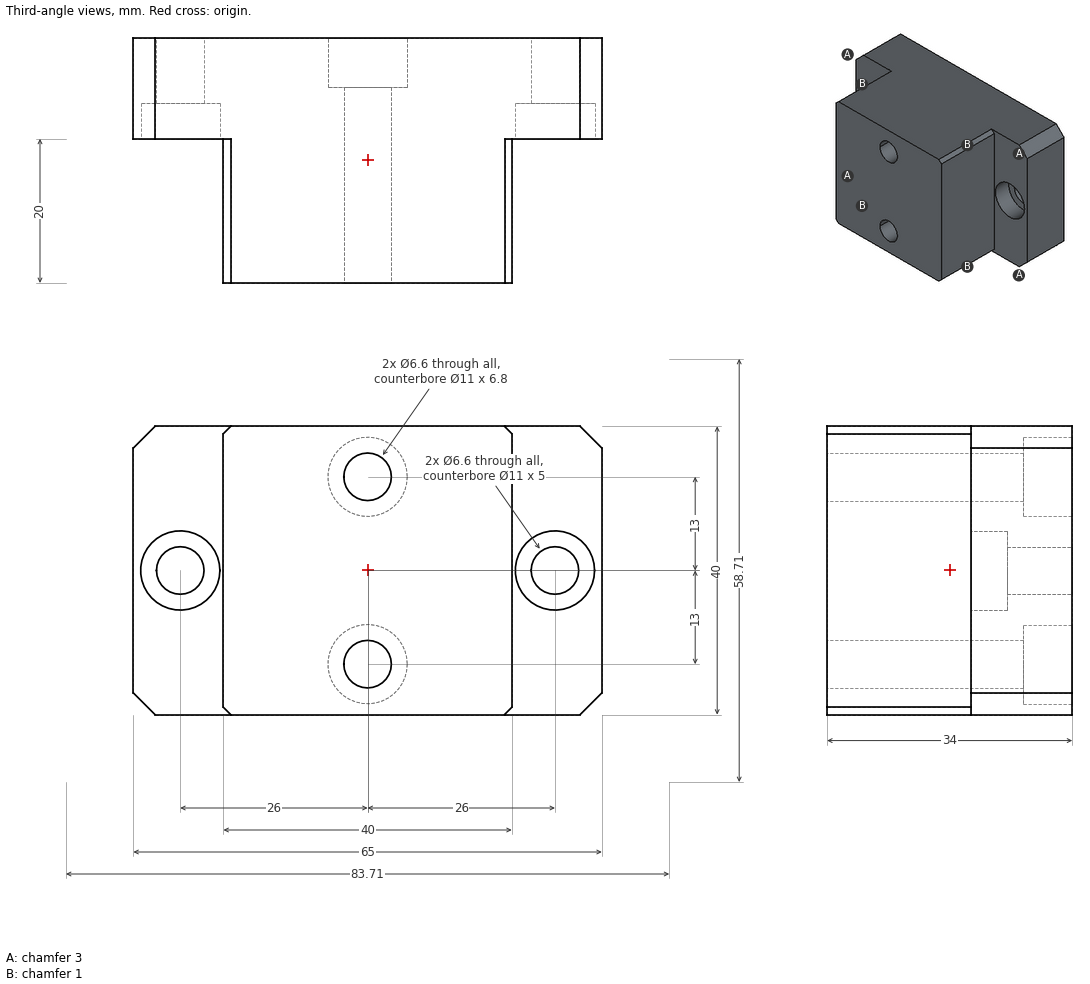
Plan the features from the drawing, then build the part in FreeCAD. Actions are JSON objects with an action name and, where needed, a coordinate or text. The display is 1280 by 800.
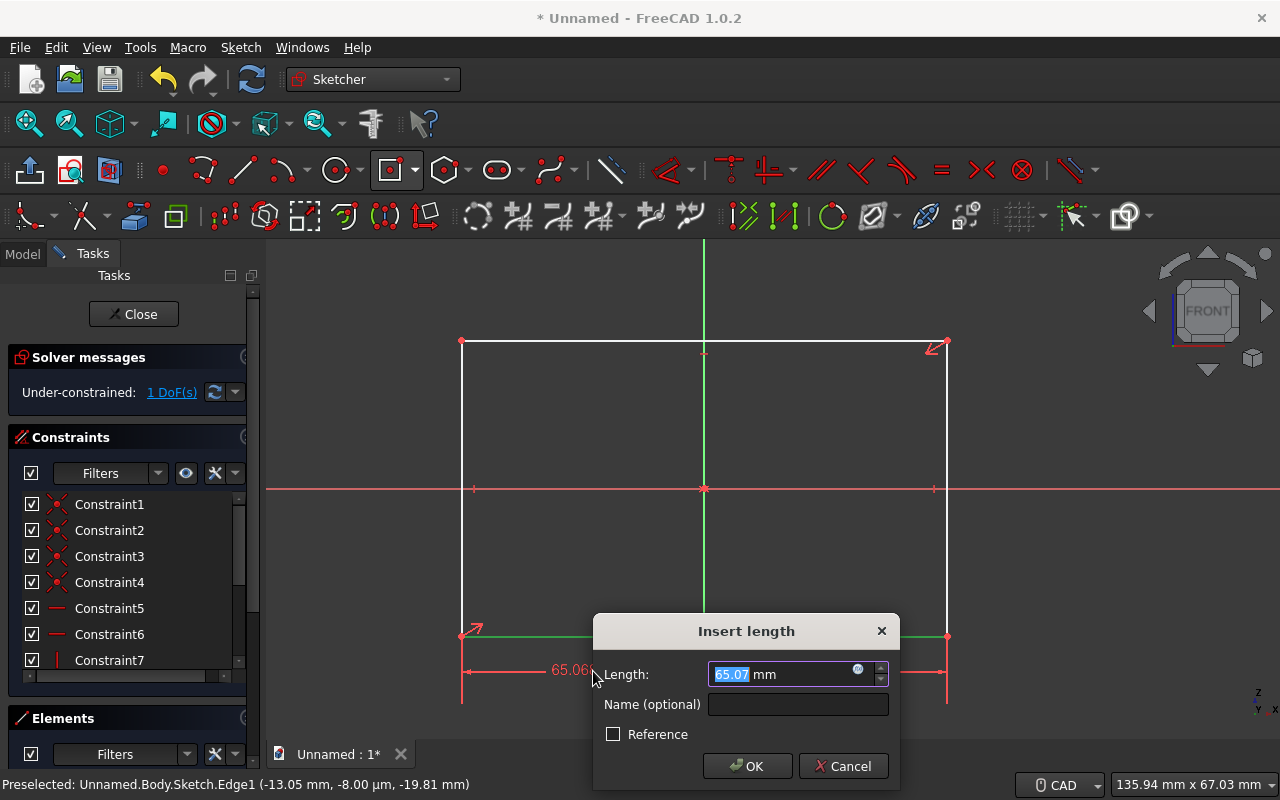
{"action": "type", "text": "65"}
{"action": "key", "text": "Return"}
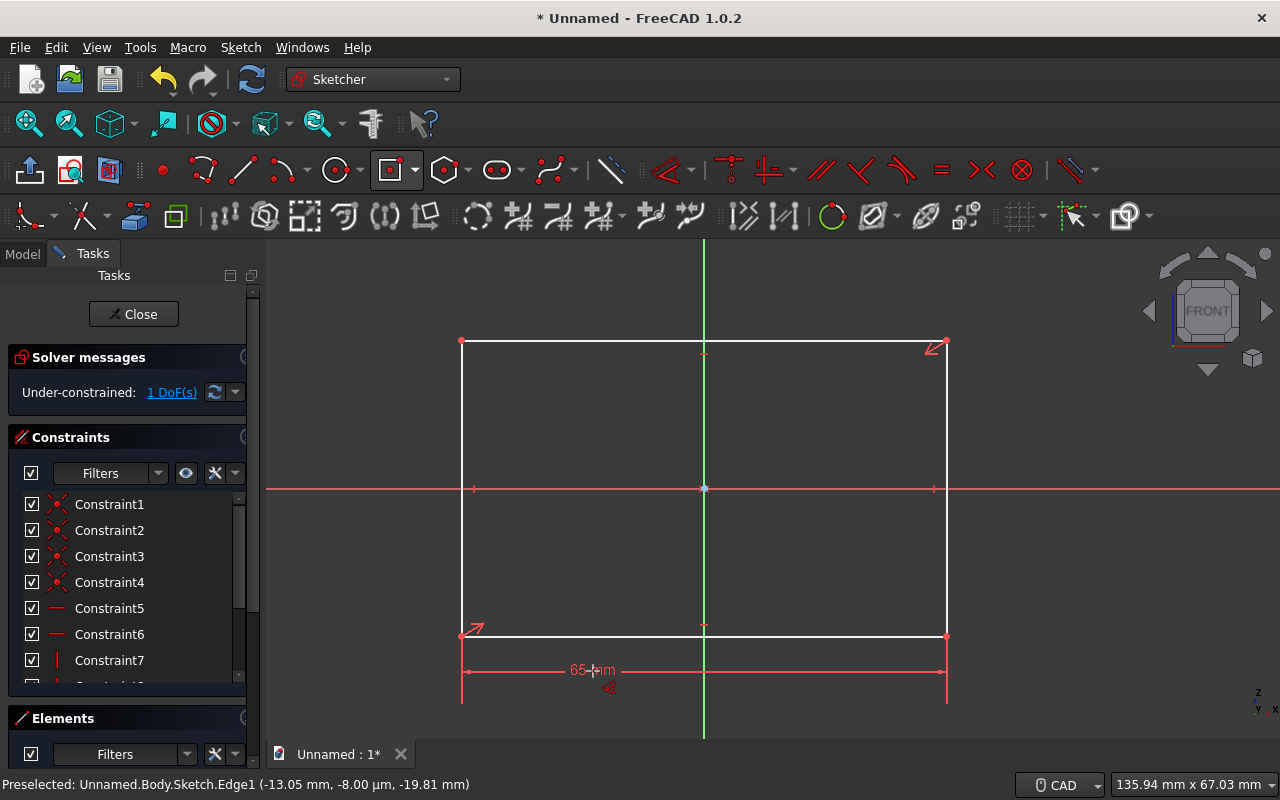
{"action": "left_click", "coordinate": [947, 548]}
{"action": "left_click", "coordinate": [981, 421]}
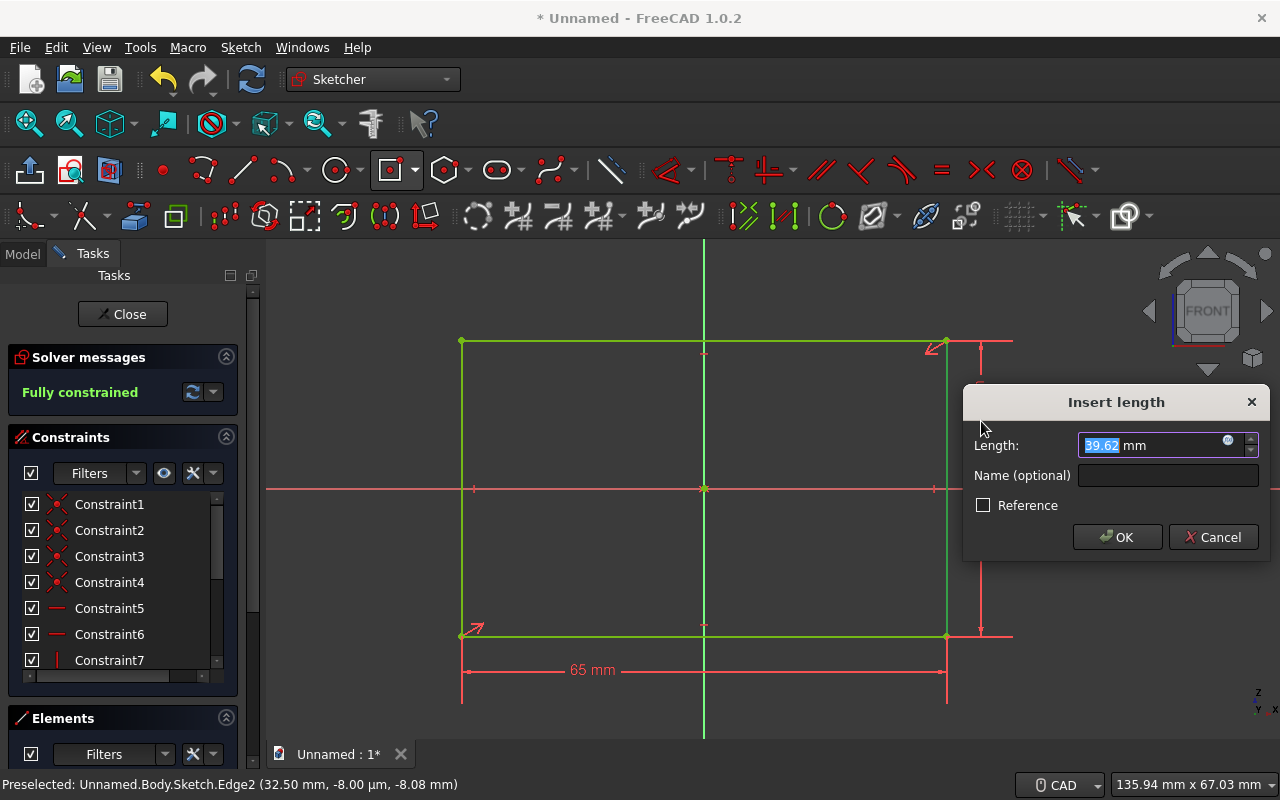
{"action": "type", "text": "40"}
{"action": "key", "text": "Return"}
{"action": "key", "text": "Escape"}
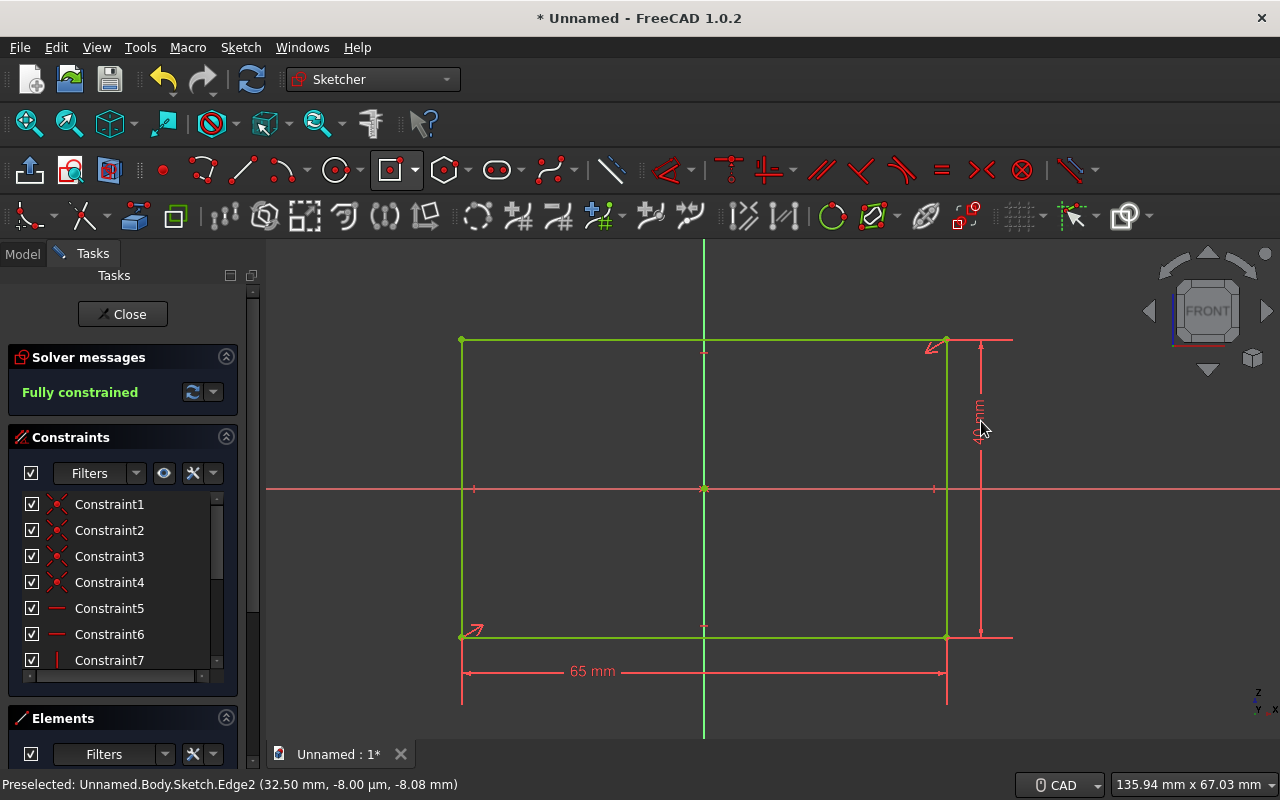
{"action": "left_click", "coordinate": [123, 314]}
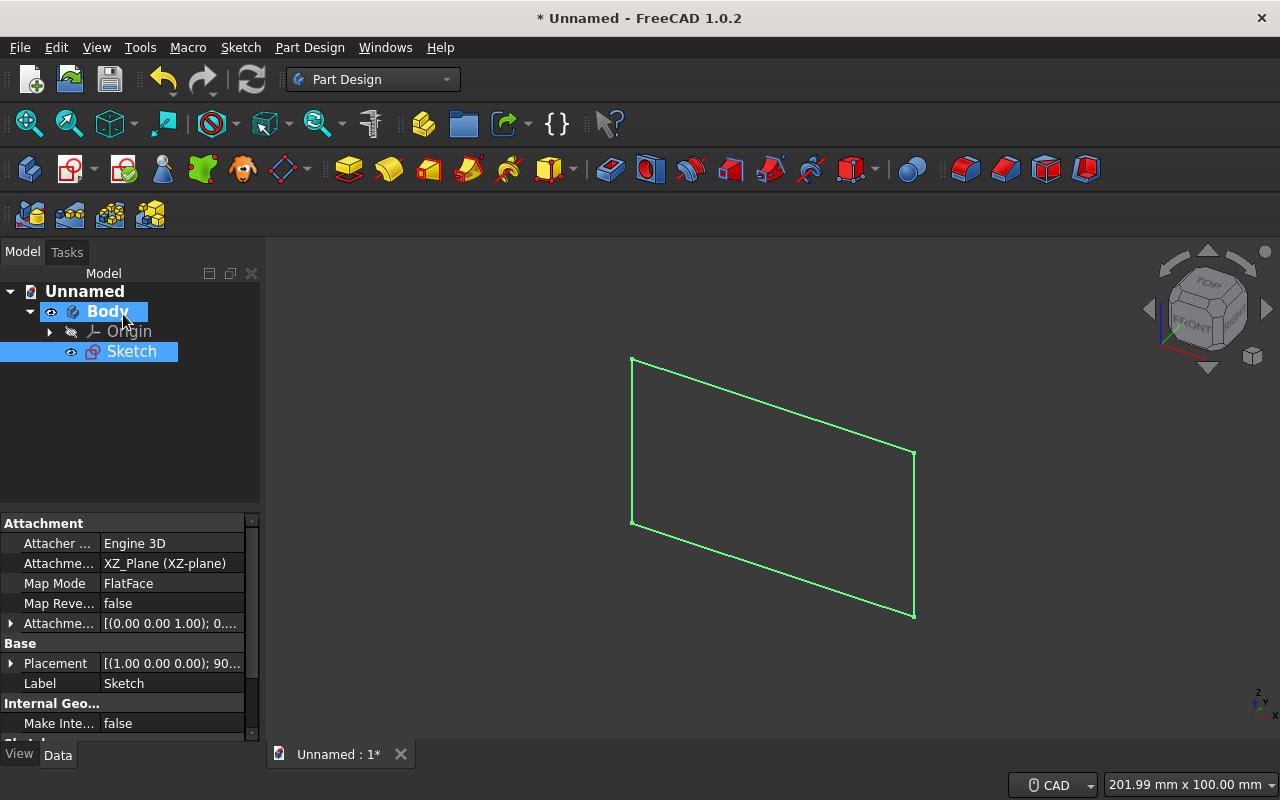
{"action": "left_click", "coordinate": [350, 170]}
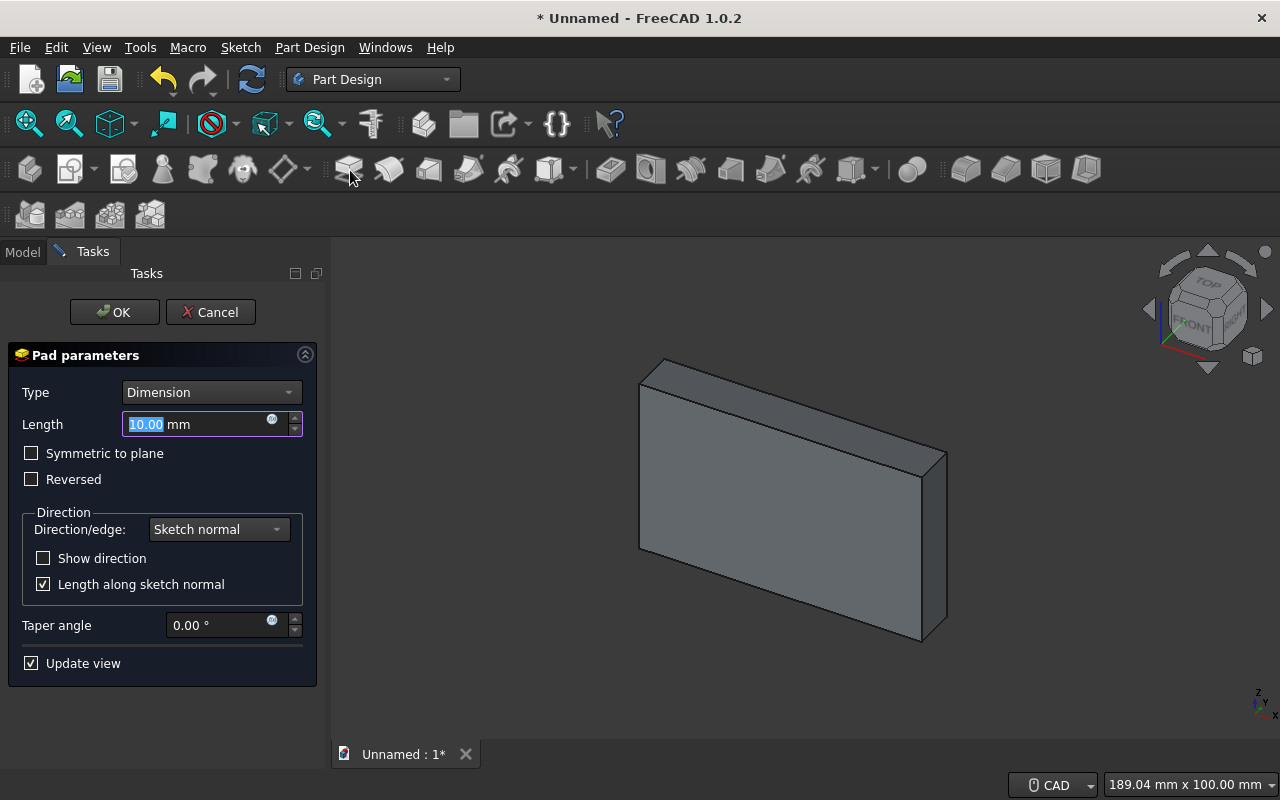
{"action": "type", "text": "34"}
{"action": "key", "text": "Tab"}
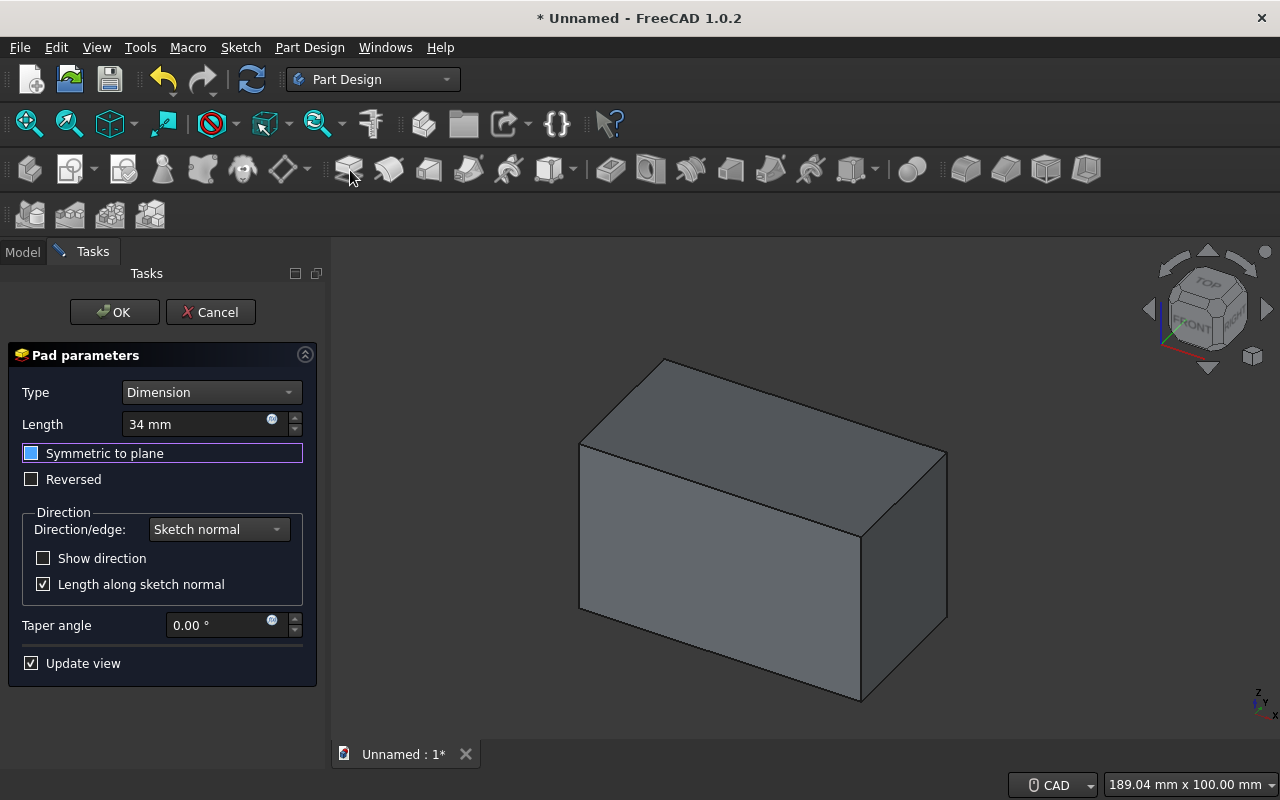
{"action": "left_click", "coordinate": [30, 453]}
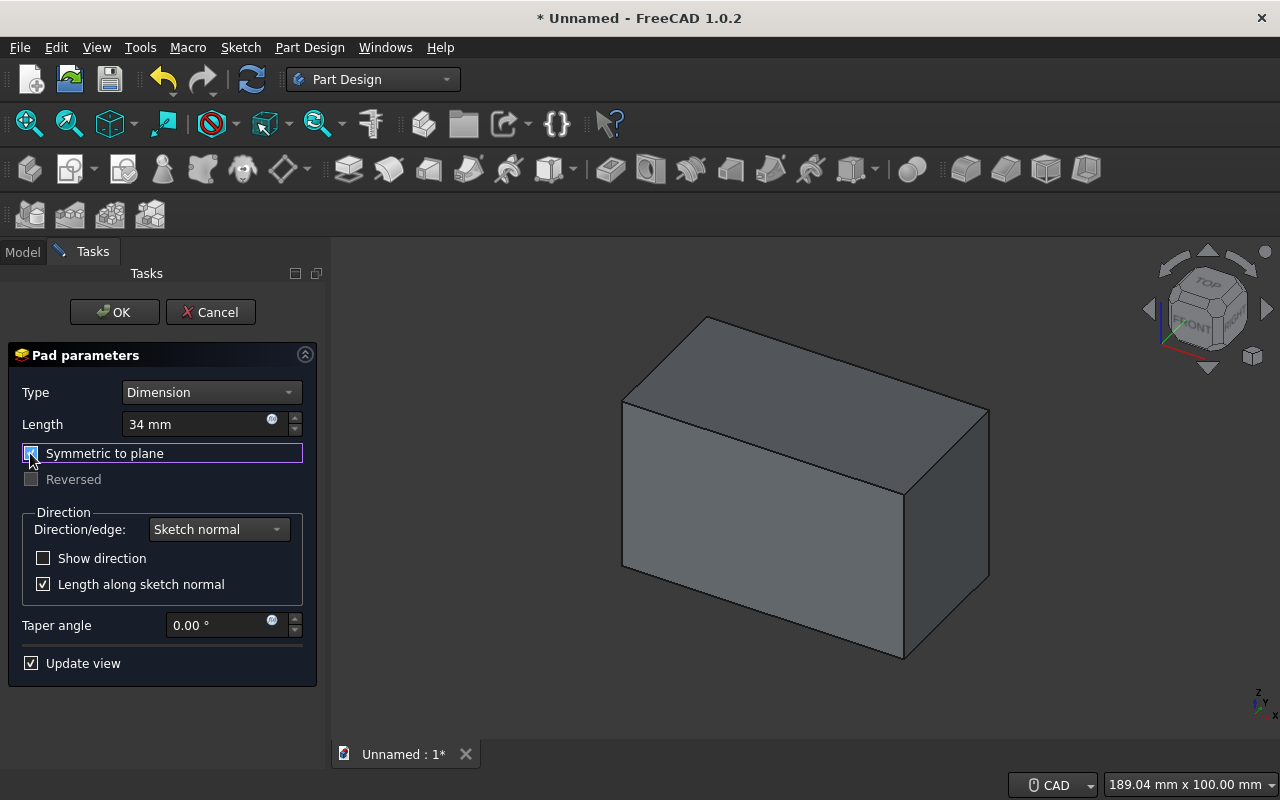
{"action": "left_click", "coordinate": [115, 312]}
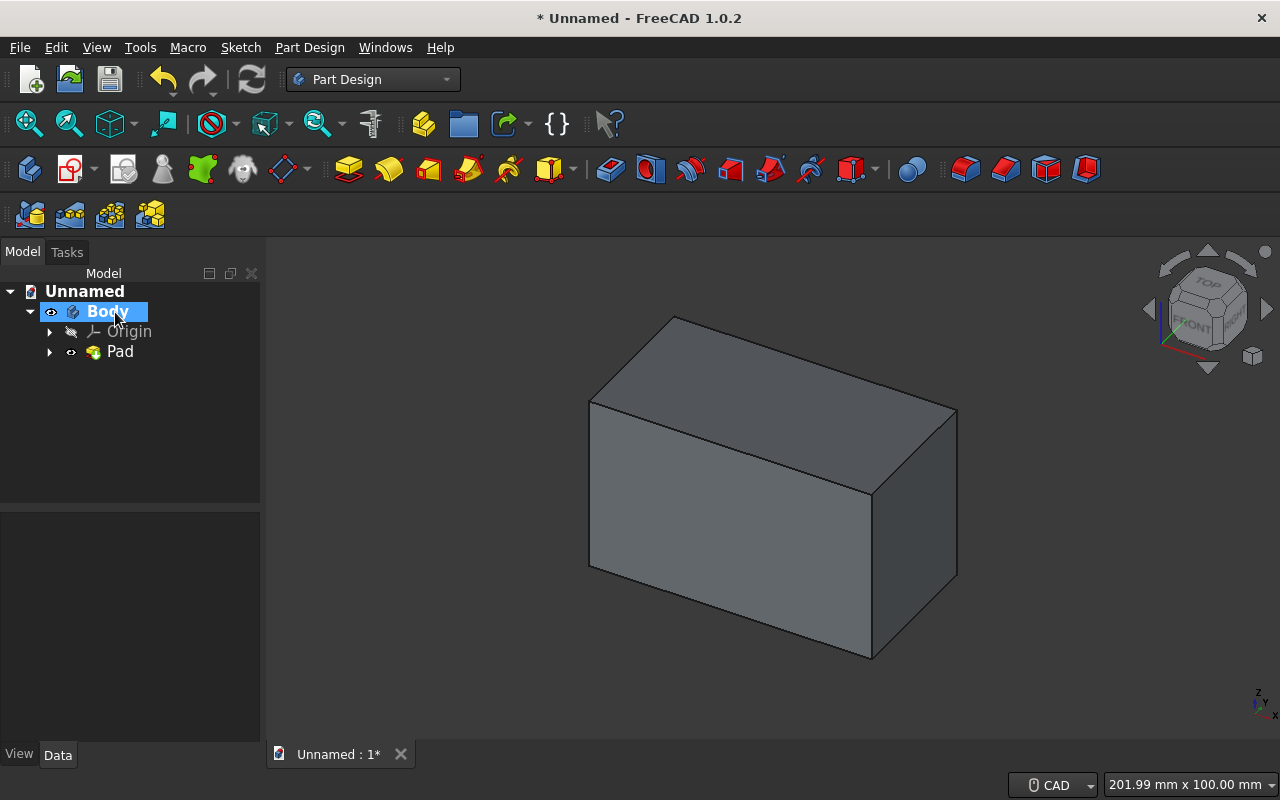
{"action": "key", "text": "4"}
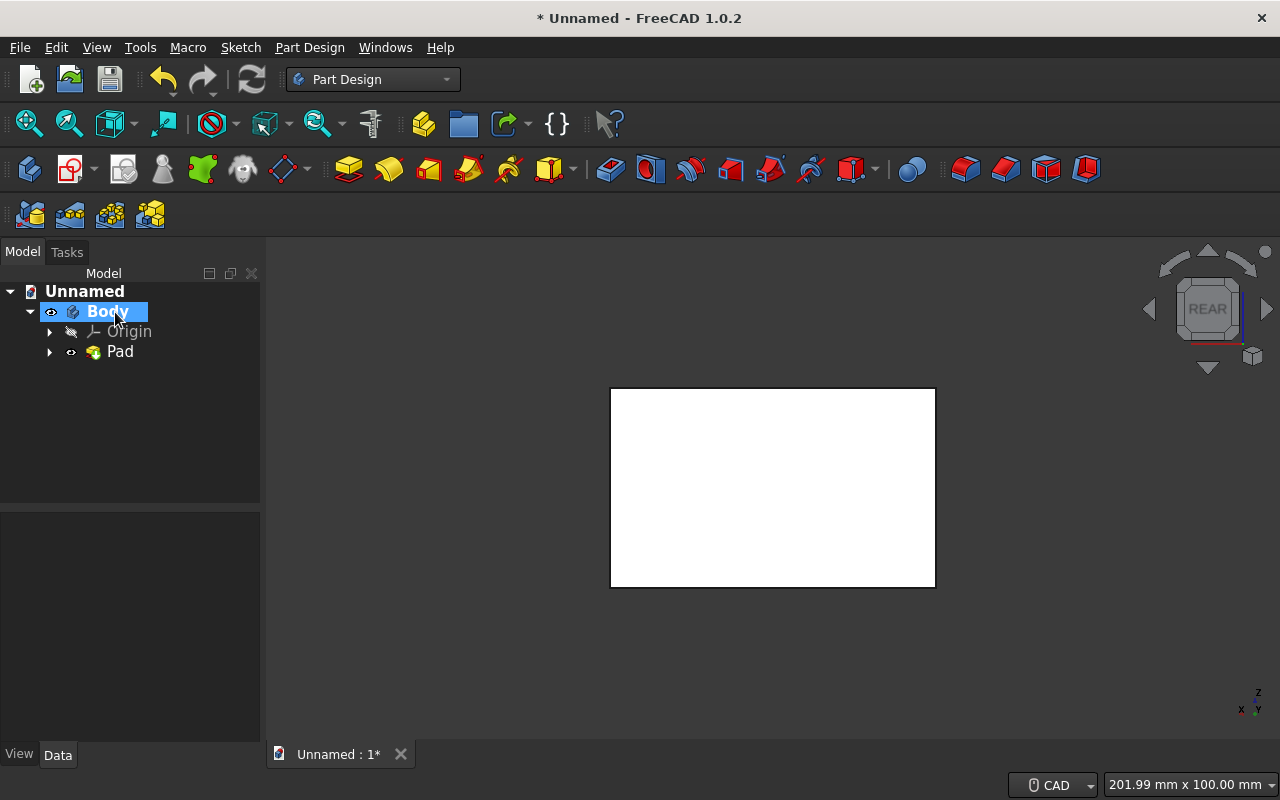
{"action": "left_click", "coordinate": [30, 124]}